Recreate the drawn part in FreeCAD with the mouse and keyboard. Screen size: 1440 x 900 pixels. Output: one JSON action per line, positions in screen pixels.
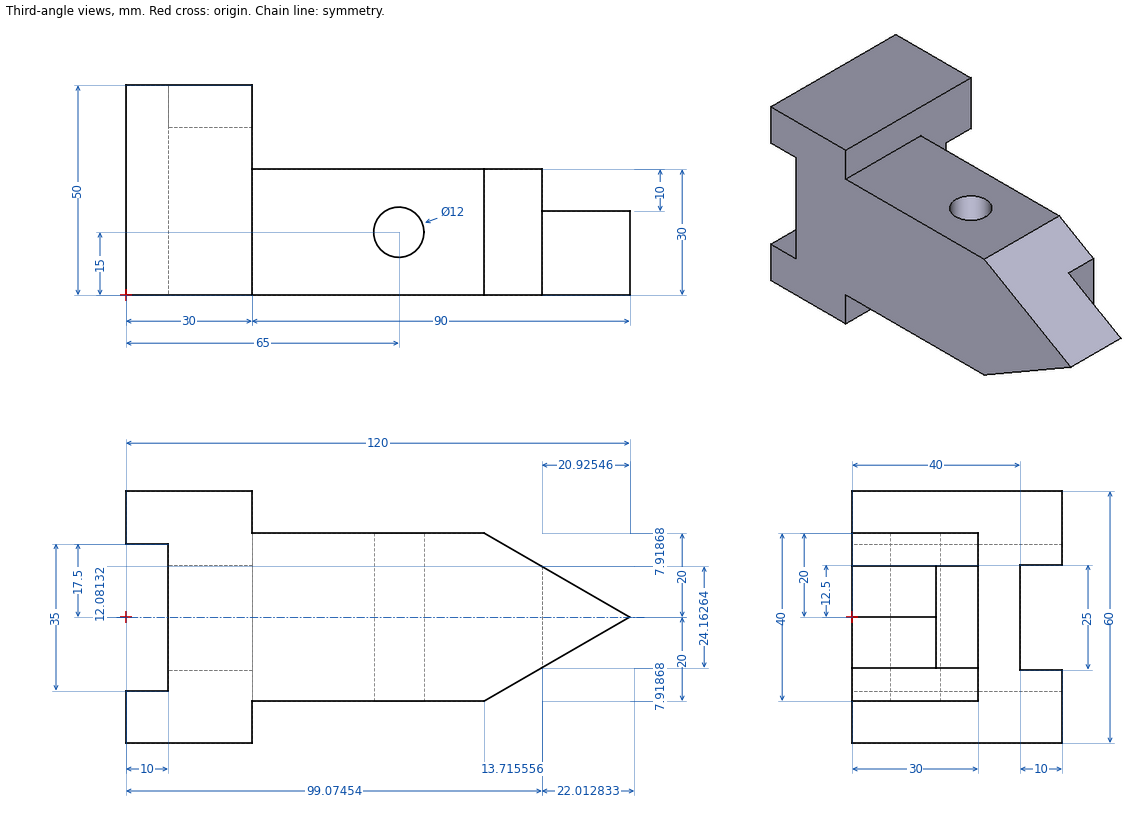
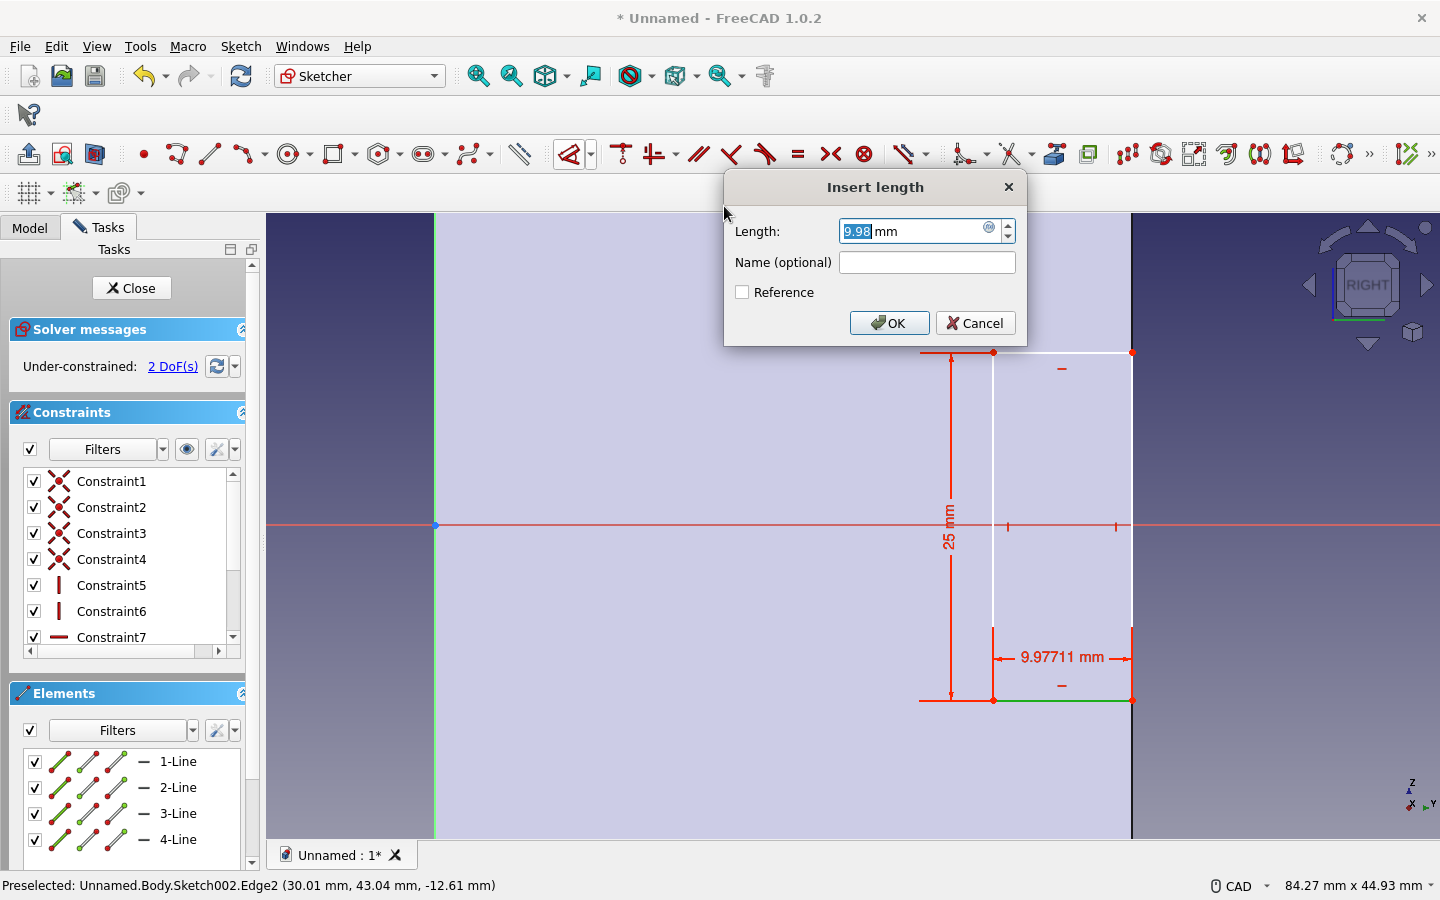
{"action": "type", "text": "10"}
{"action": "key", "text": "Return"}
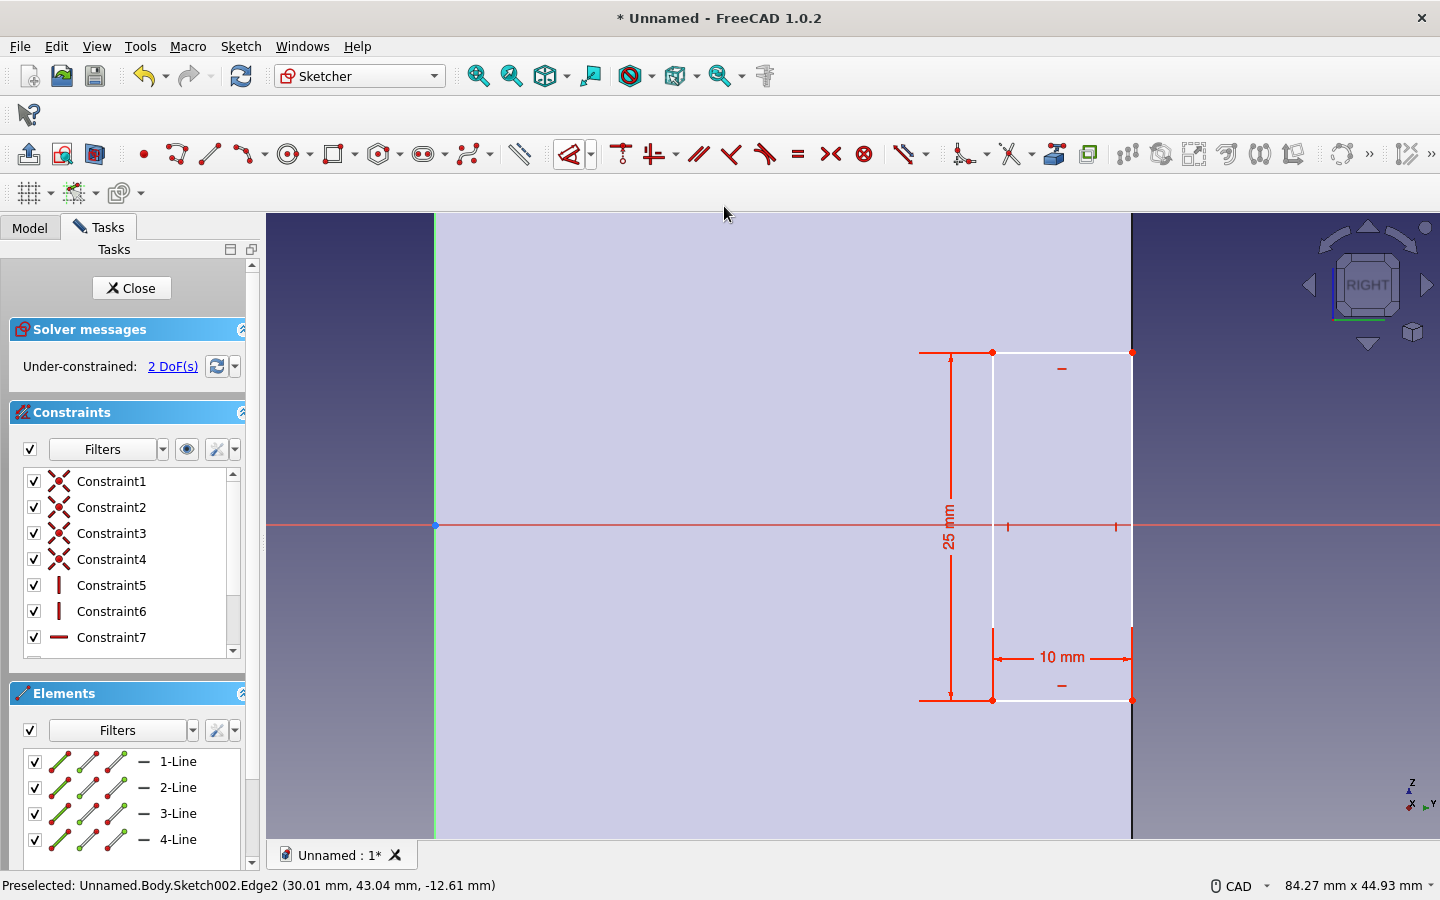
{"action": "left_click", "coordinate": [993, 353]}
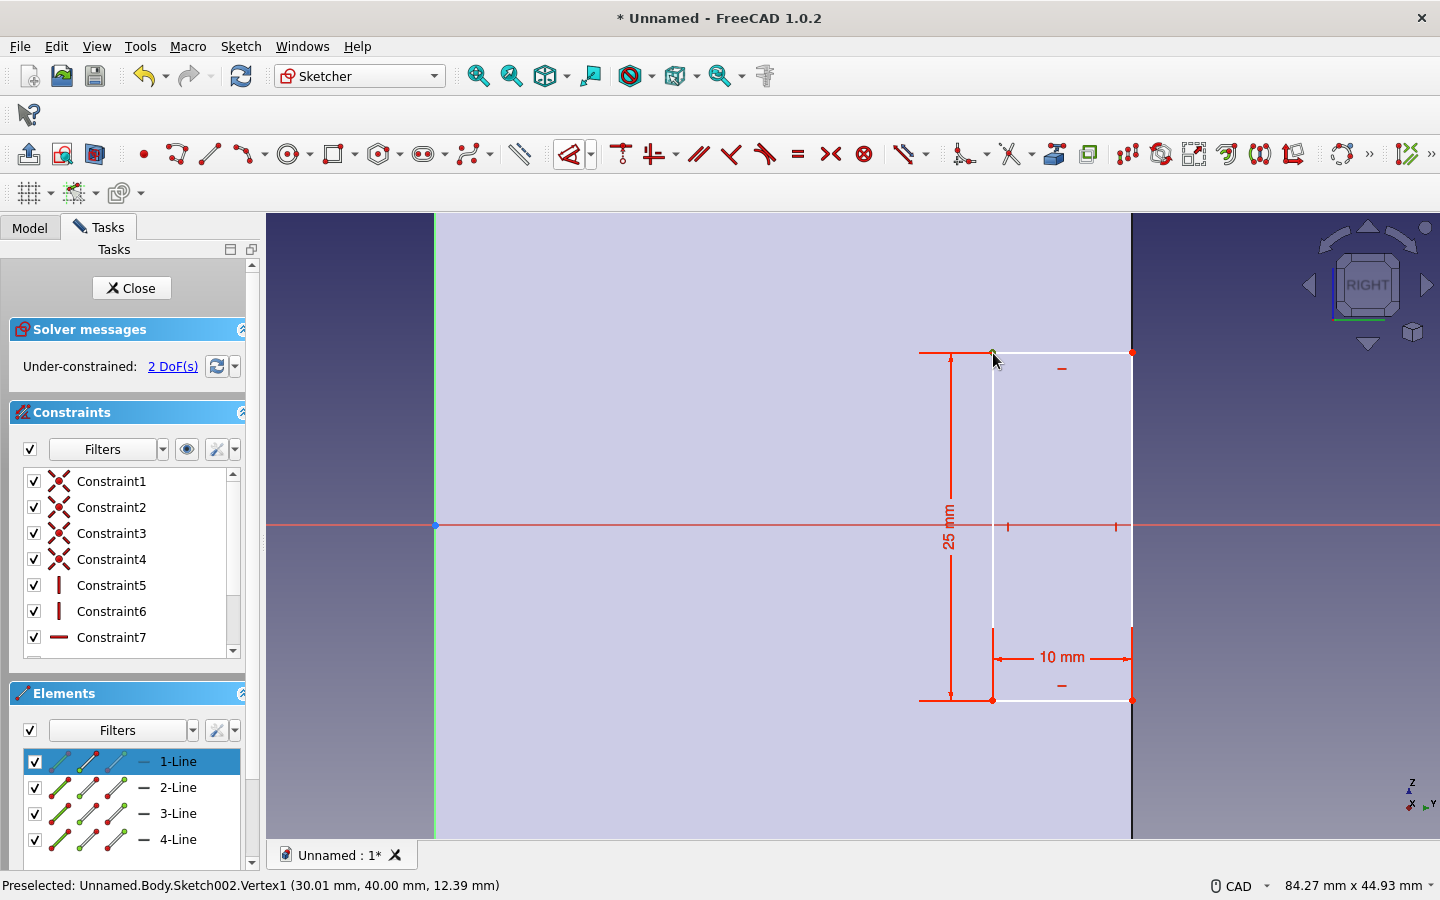
{"action": "key", "text": "l"}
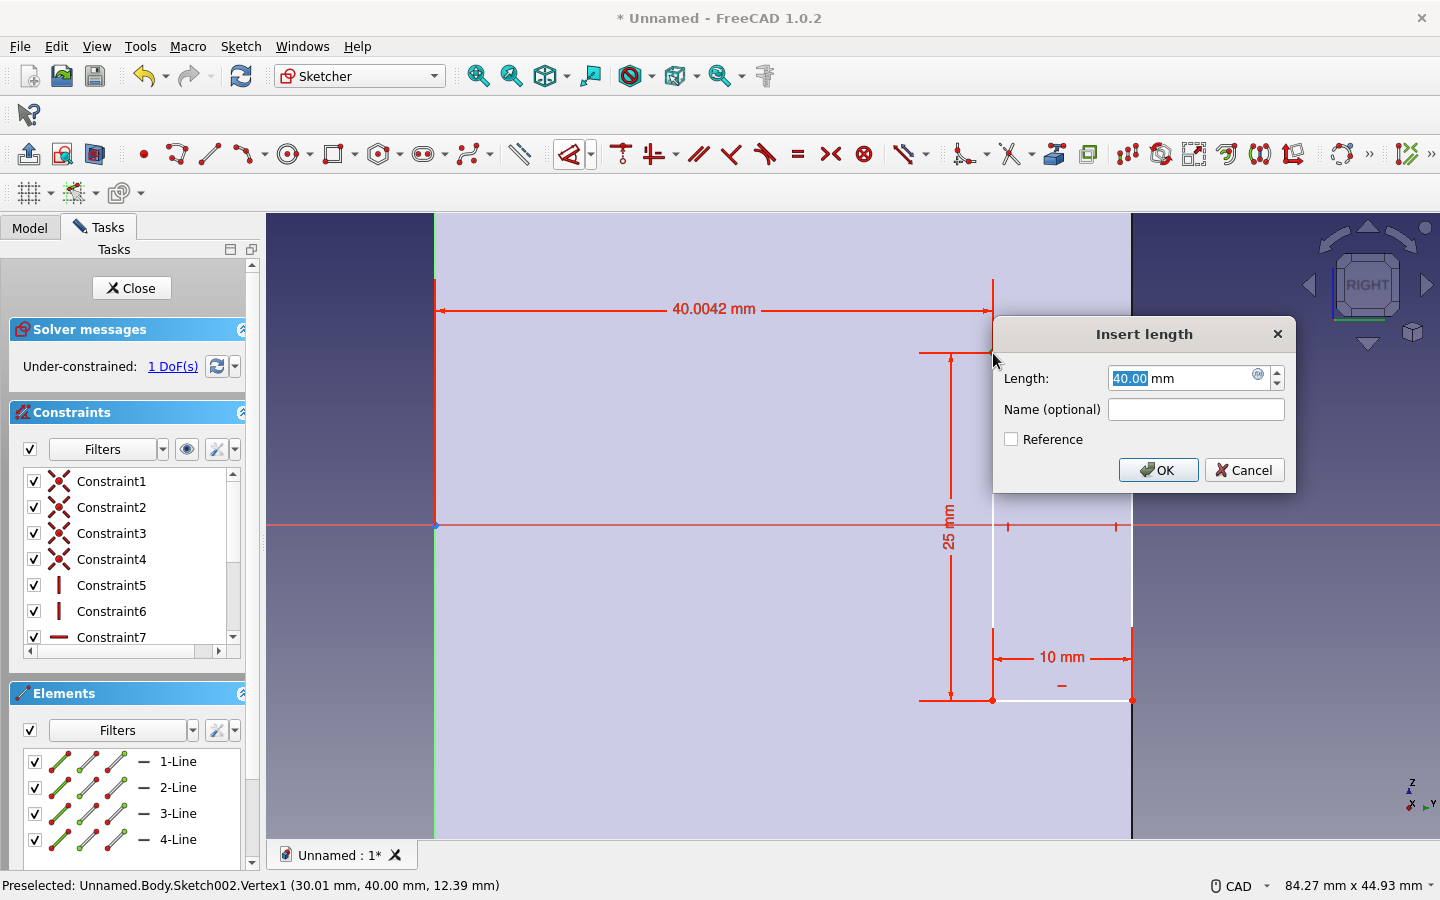
{"action": "type", "text": "40"}
{"action": "key", "text": "Return"}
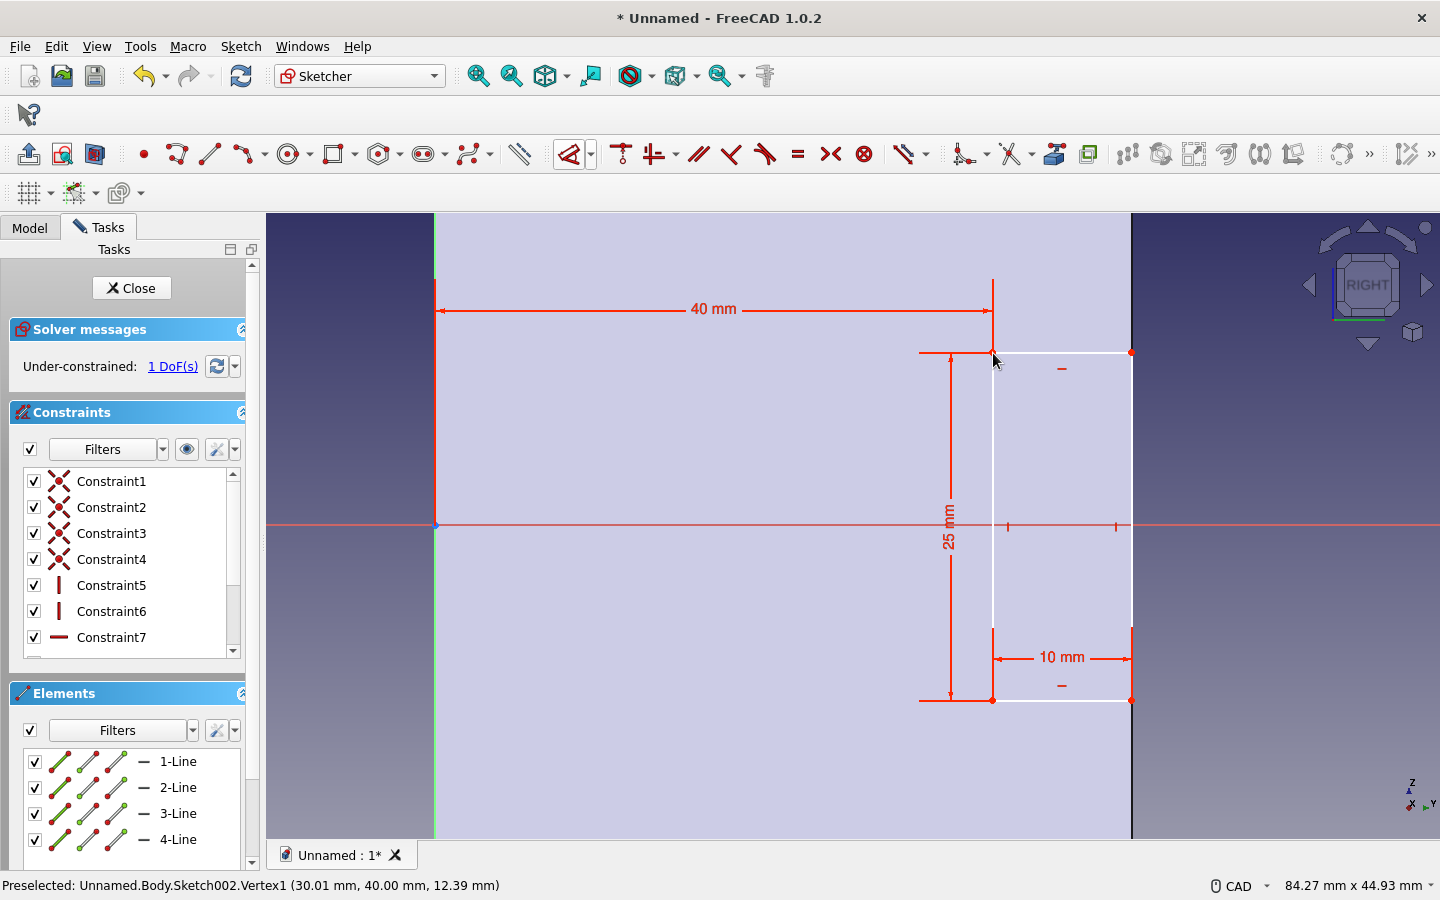
{"action": "left_click", "coordinate": [993, 353]}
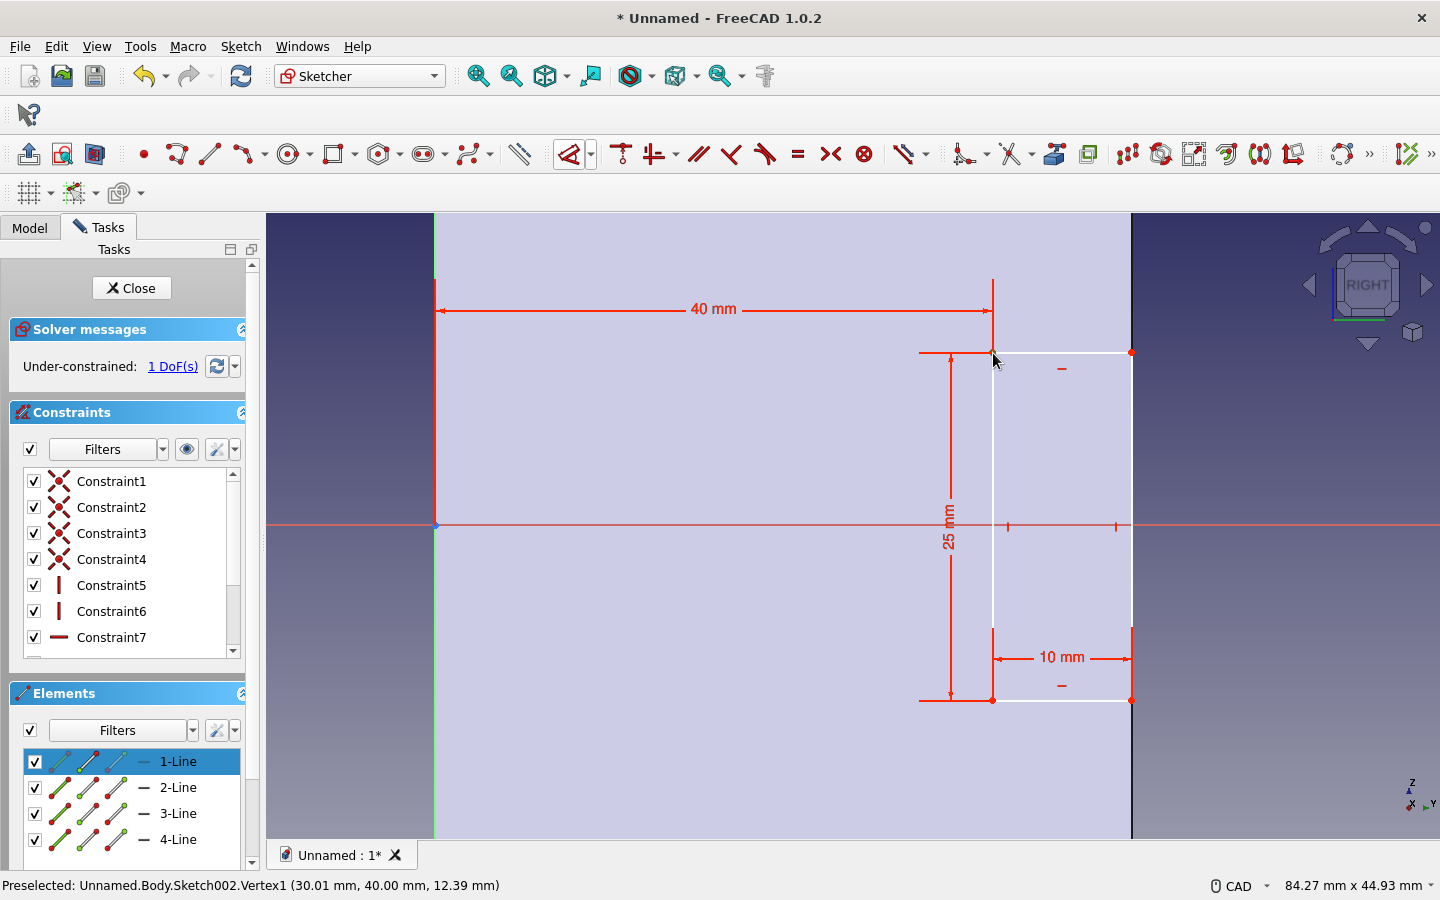
{"action": "key", "text": "i"}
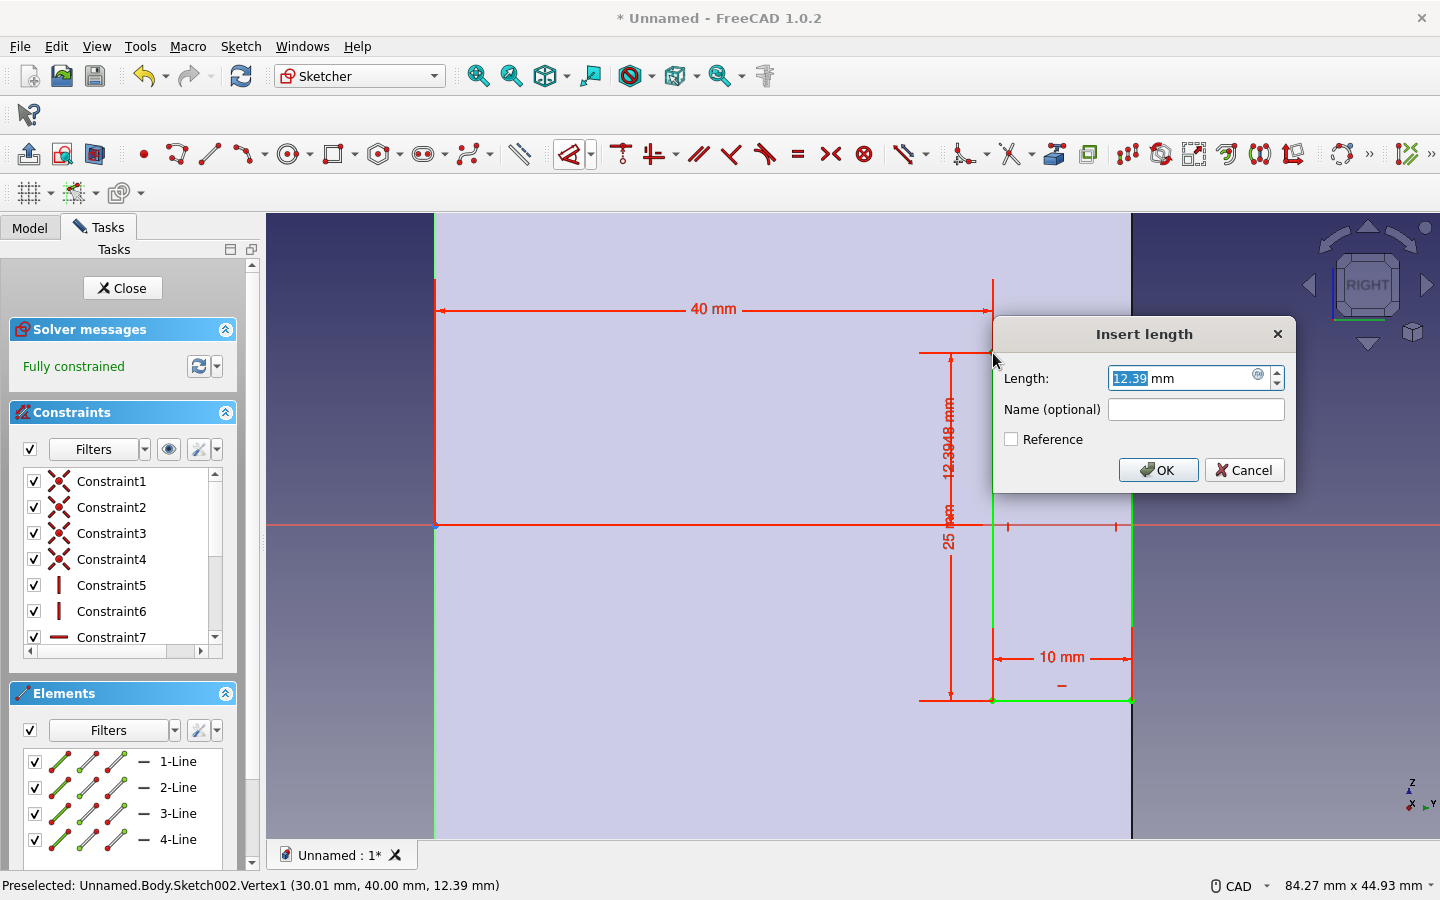
{"action": "type", "text": "12.5"}
{"action": "key", "text": "Return"}